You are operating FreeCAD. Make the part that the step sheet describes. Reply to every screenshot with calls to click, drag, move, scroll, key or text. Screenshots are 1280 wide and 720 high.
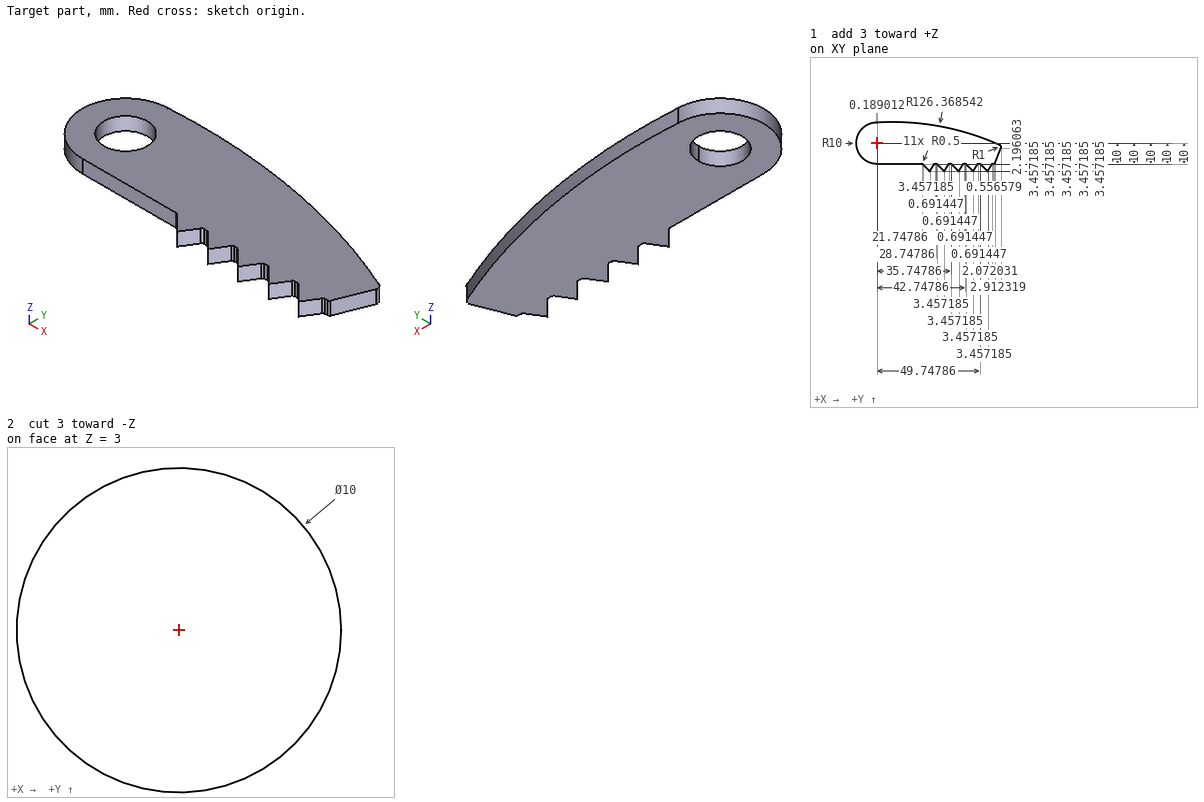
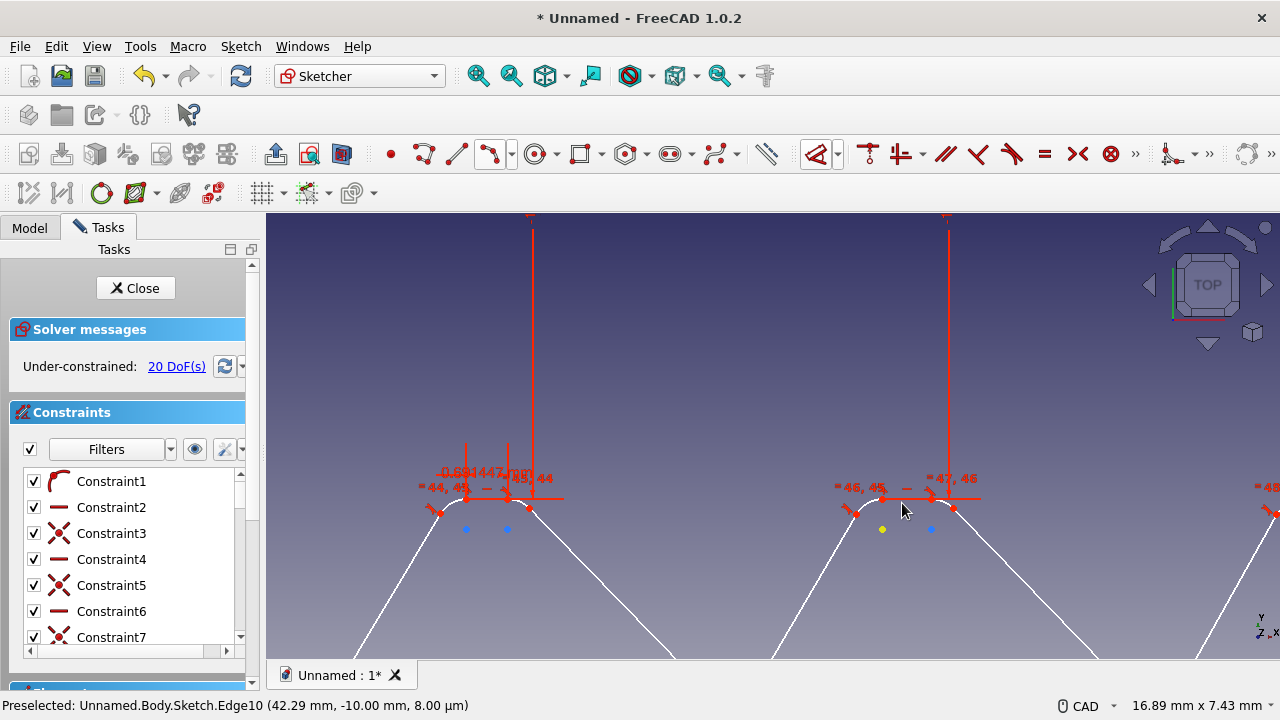
click(897, 499)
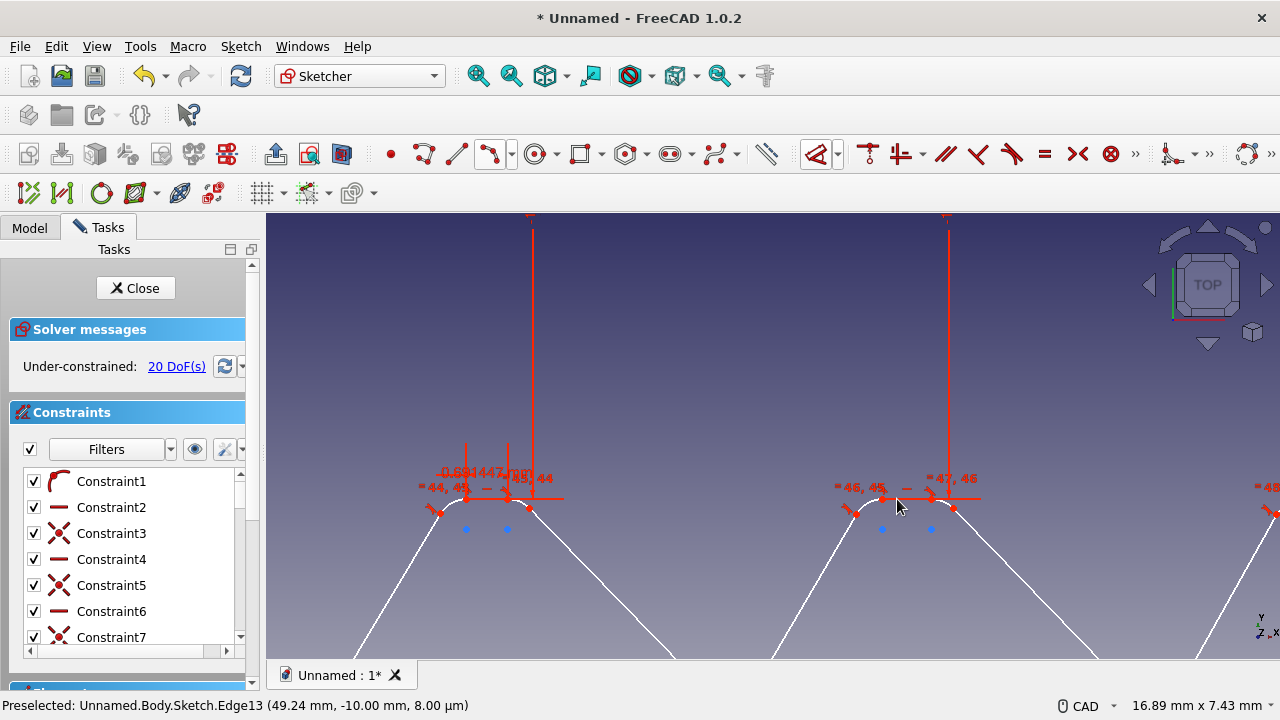
key(l)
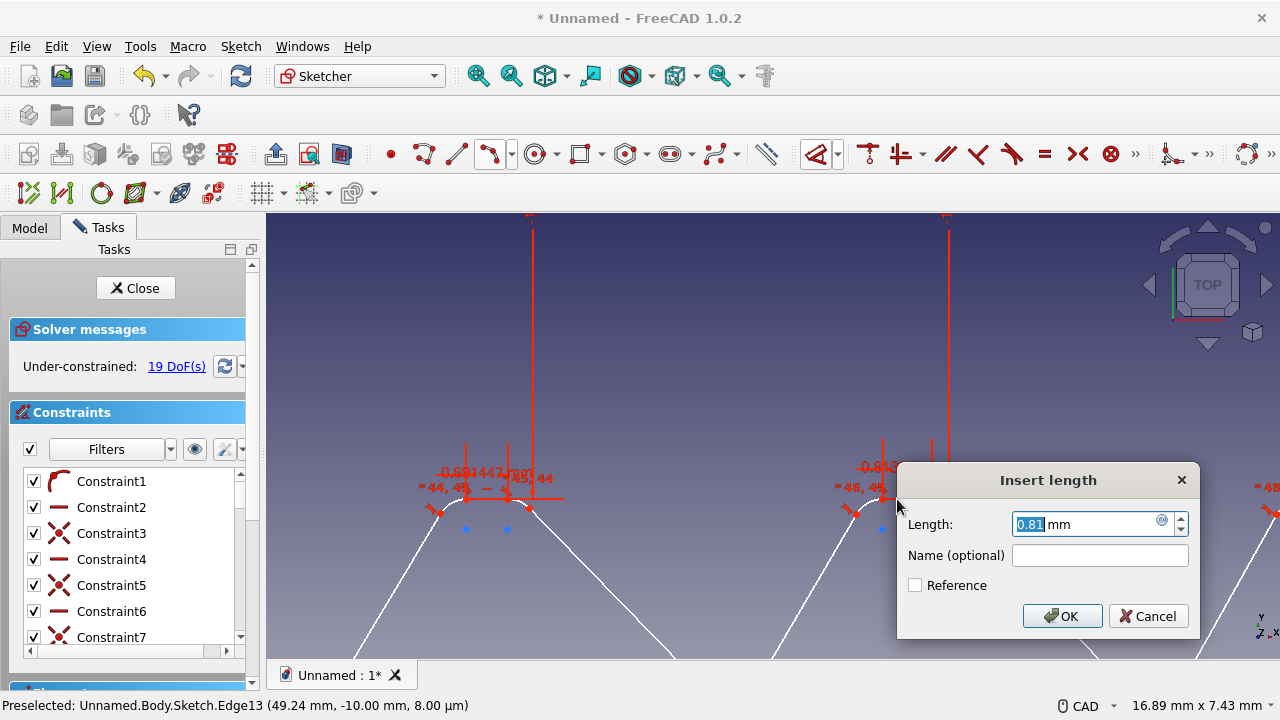
text(0.691447)
key(Return)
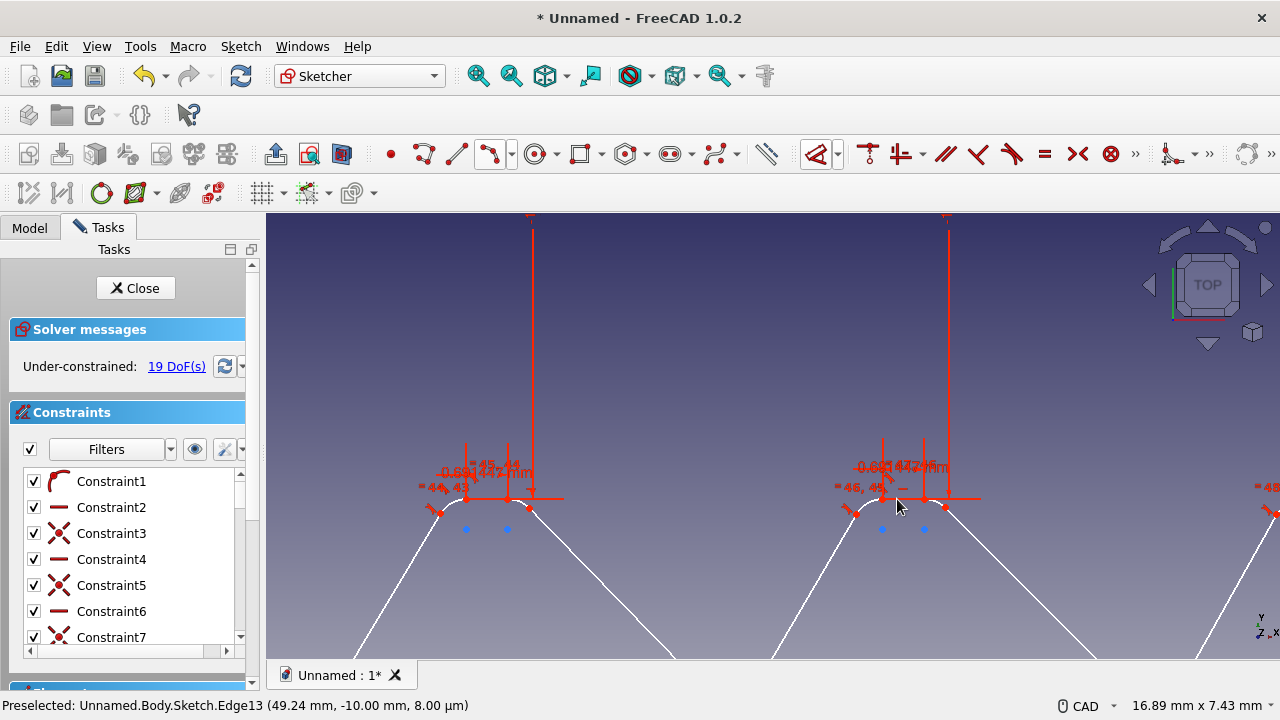
scroll(902, 503, down, 10)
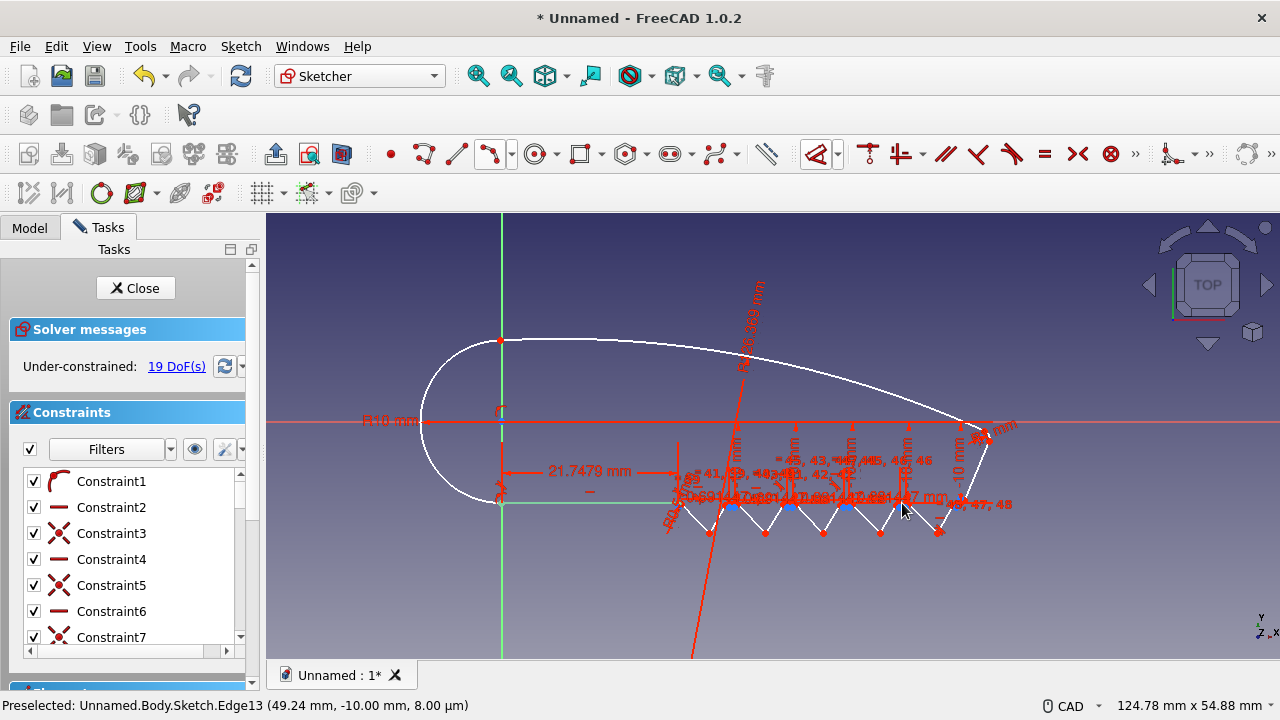
scroll(958, 503, up, 11)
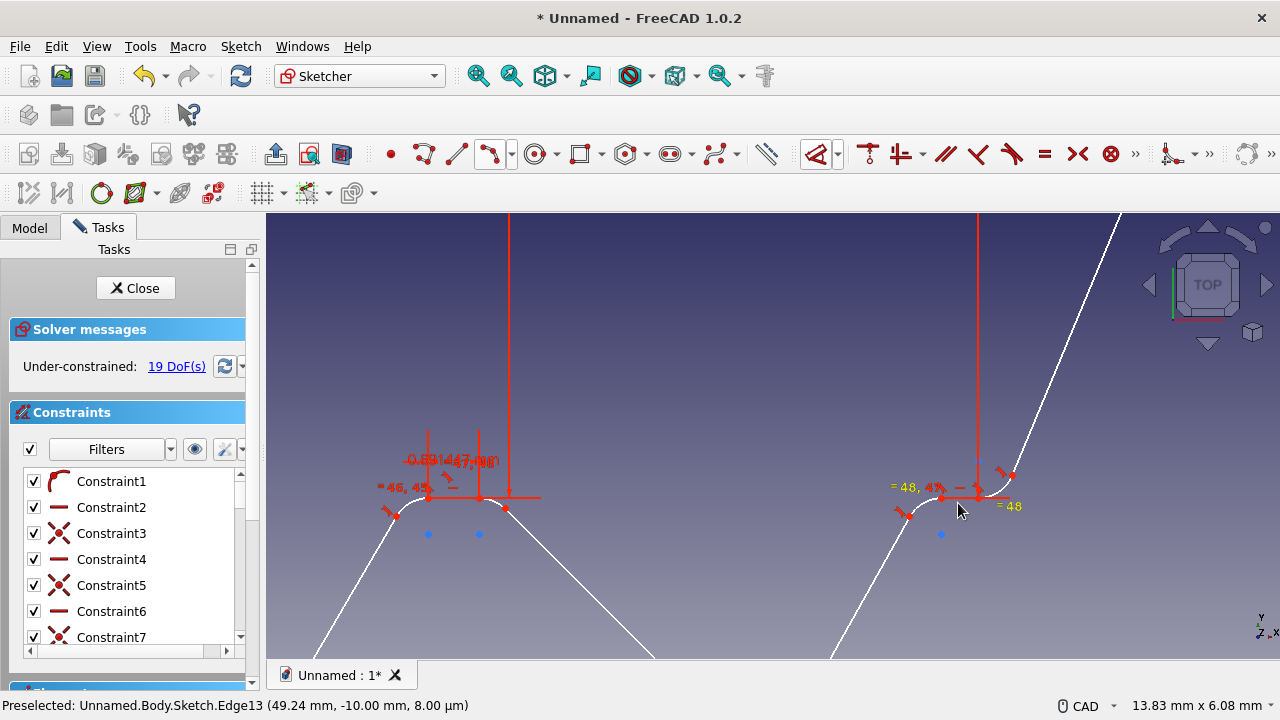
click(956, 498)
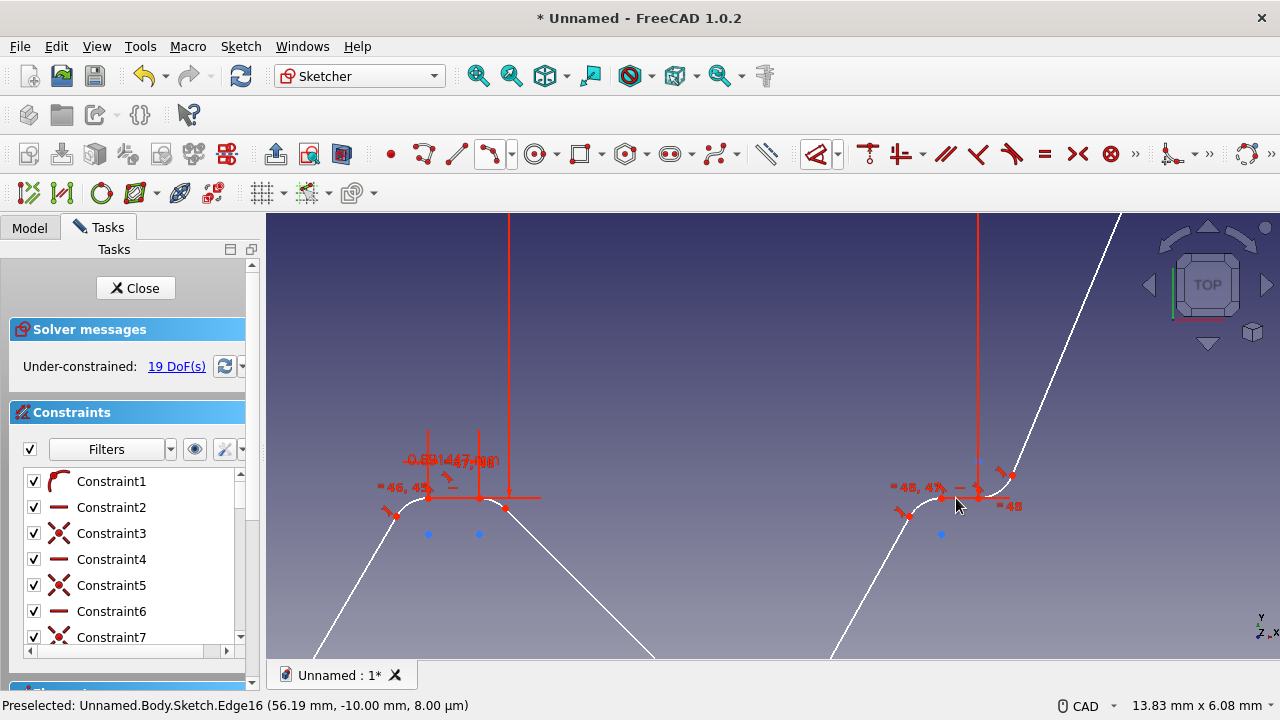
click(838, 154)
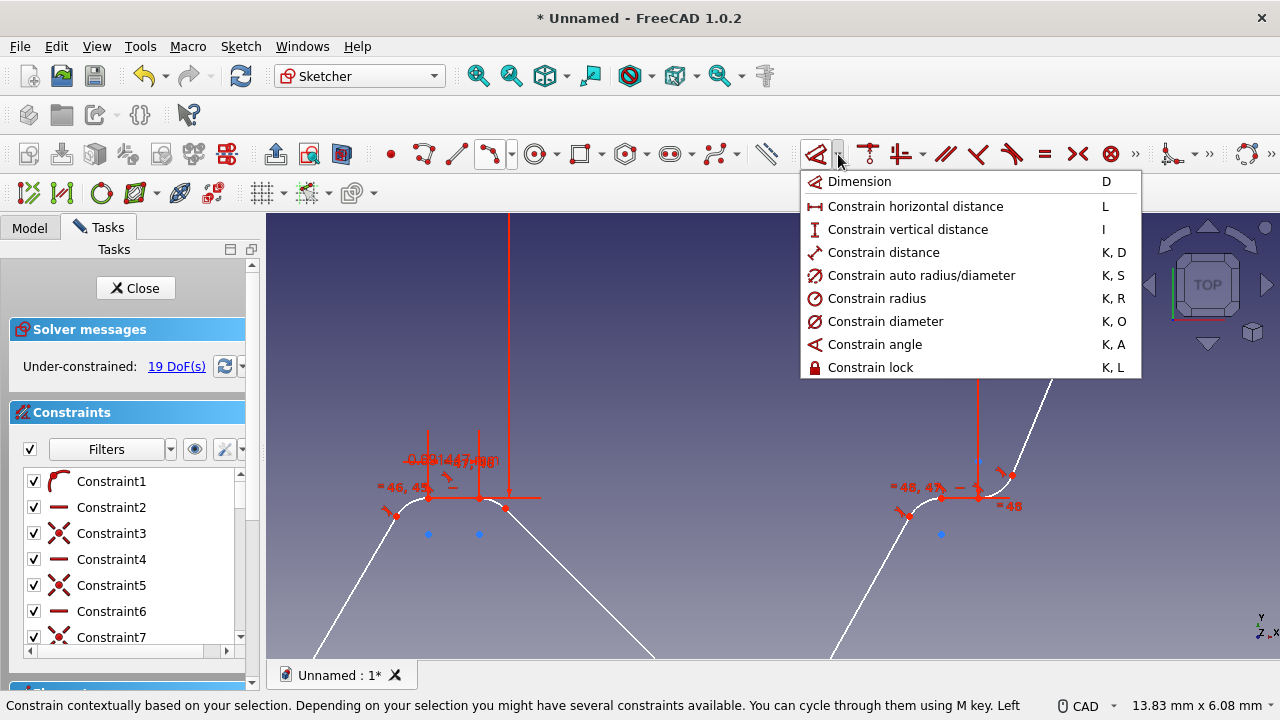
click(971, 206)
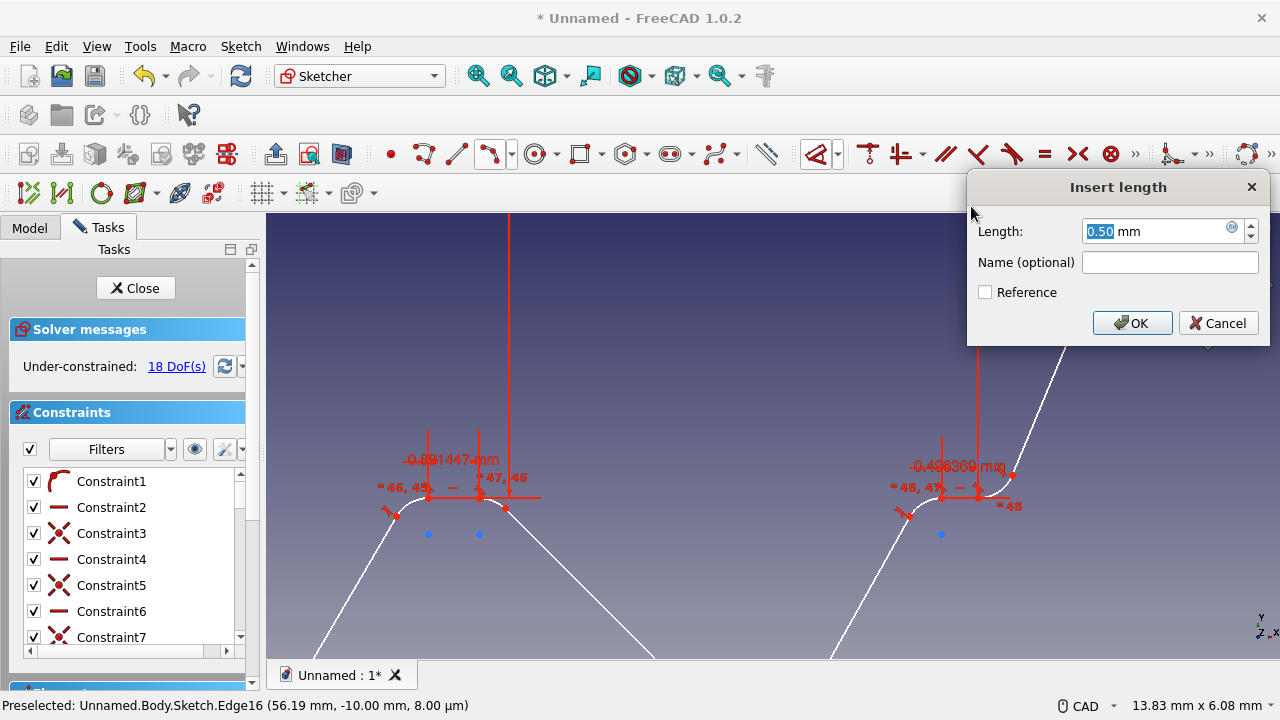
text(0.556579)
key(Return)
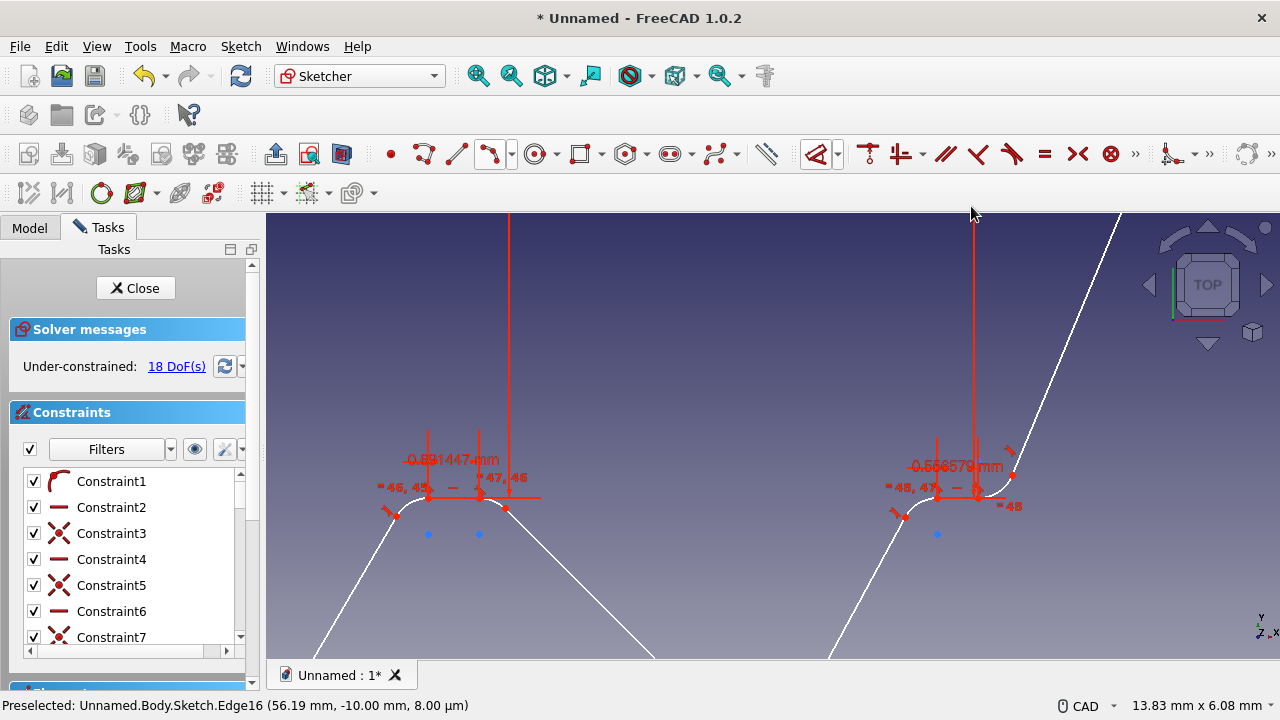
scroll(958, 503, down, 11)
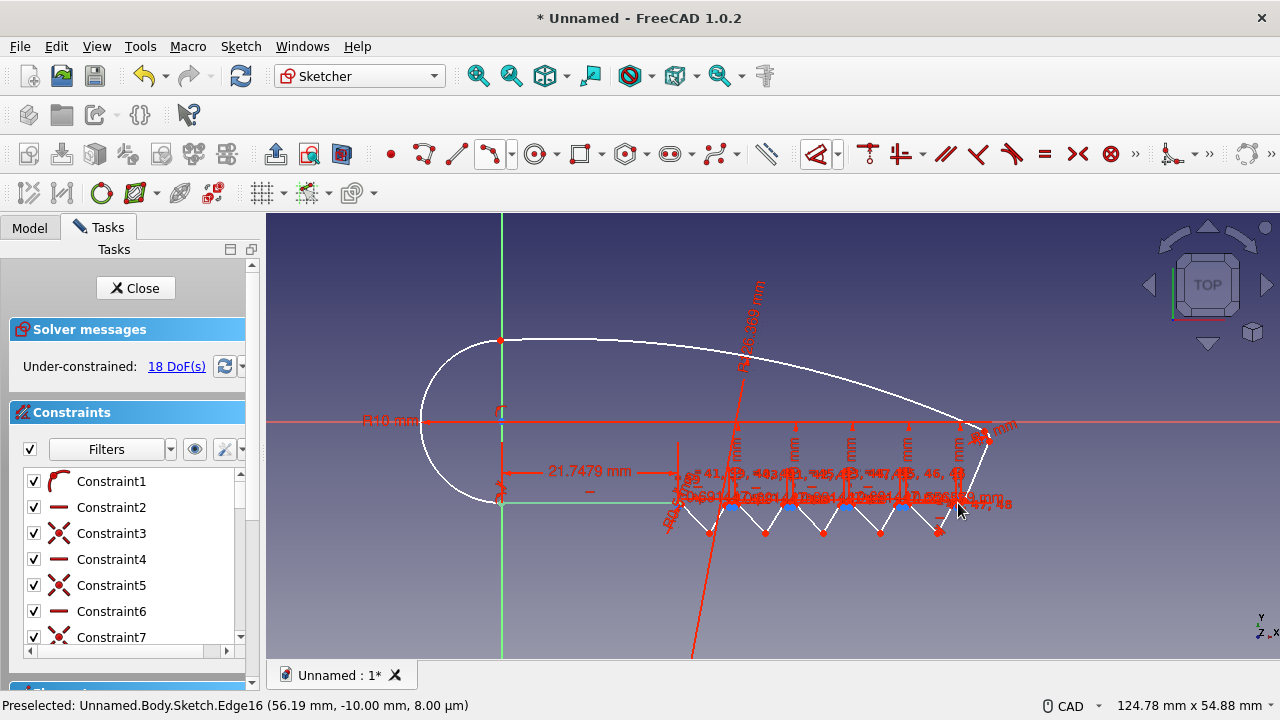
scroll(735, 503, up, 7)